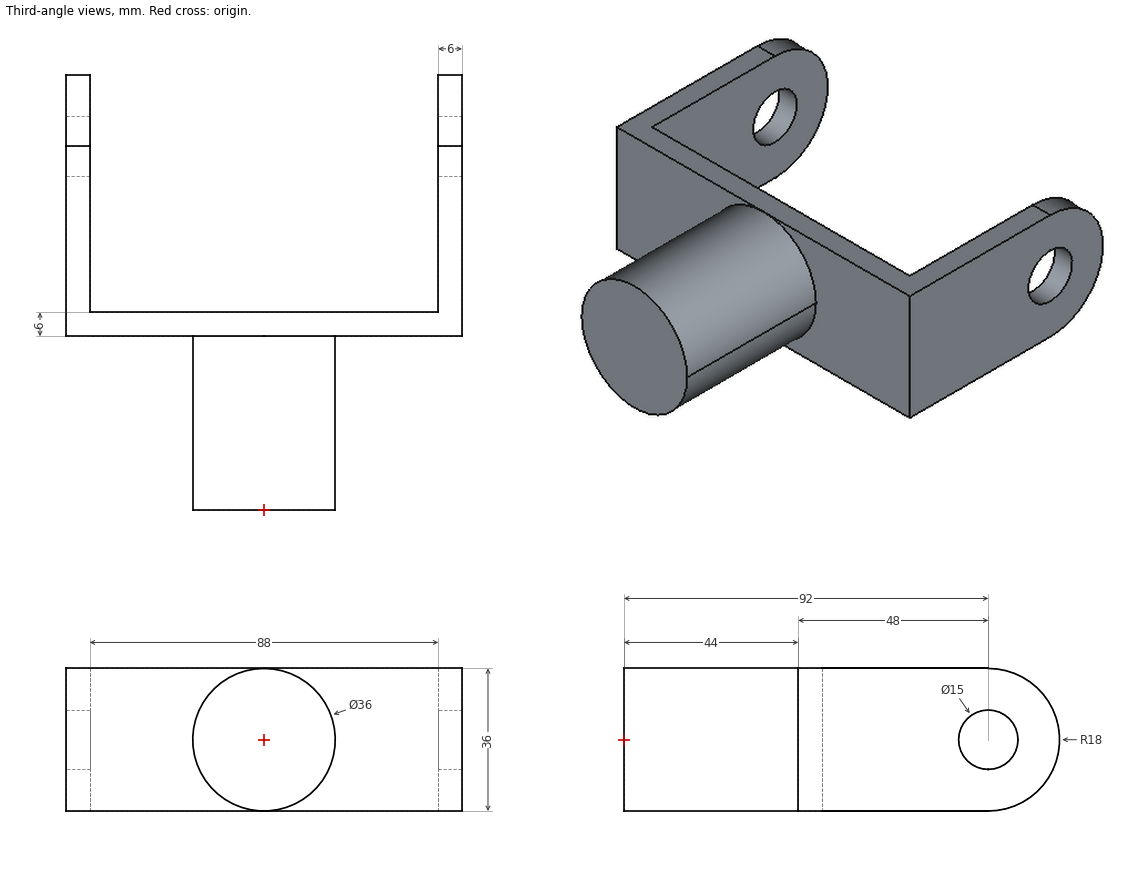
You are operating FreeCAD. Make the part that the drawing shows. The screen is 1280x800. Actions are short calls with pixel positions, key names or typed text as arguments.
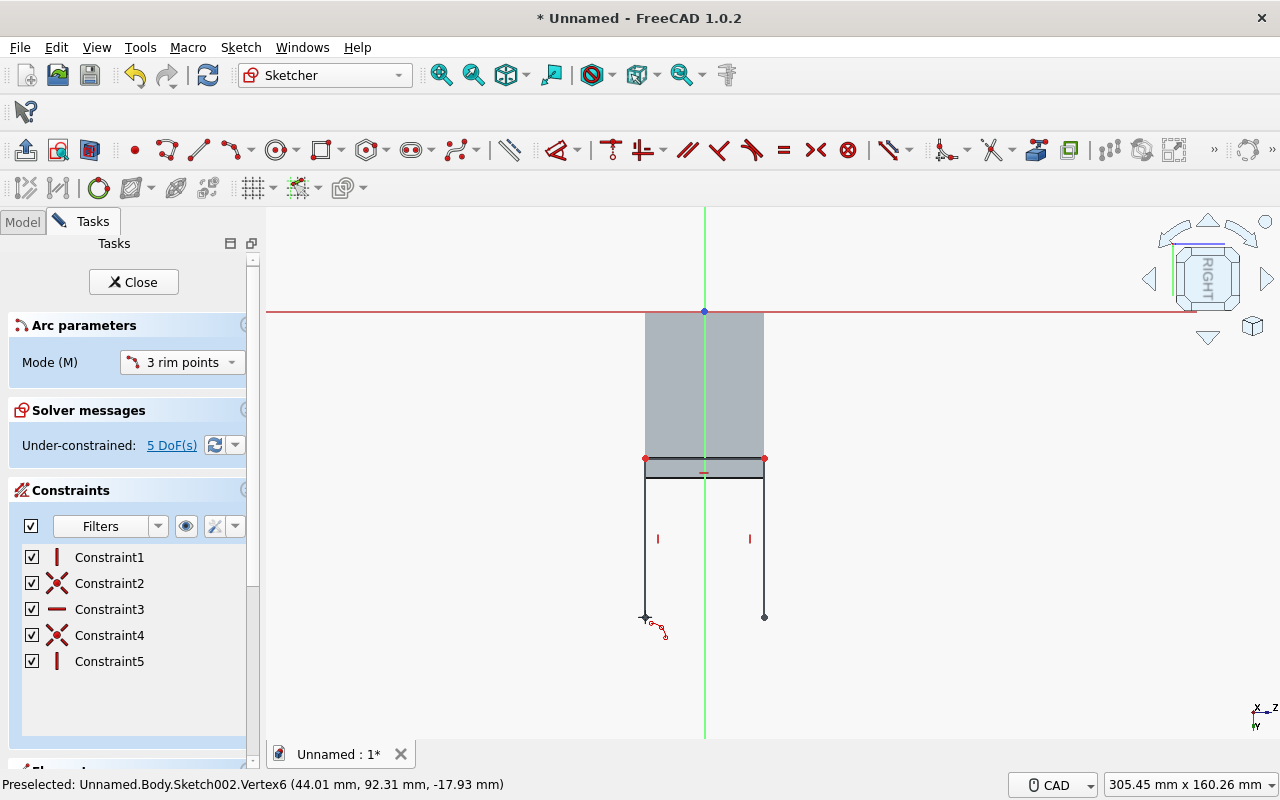
click(645, 618)
click(764, 618)
click(686, 674)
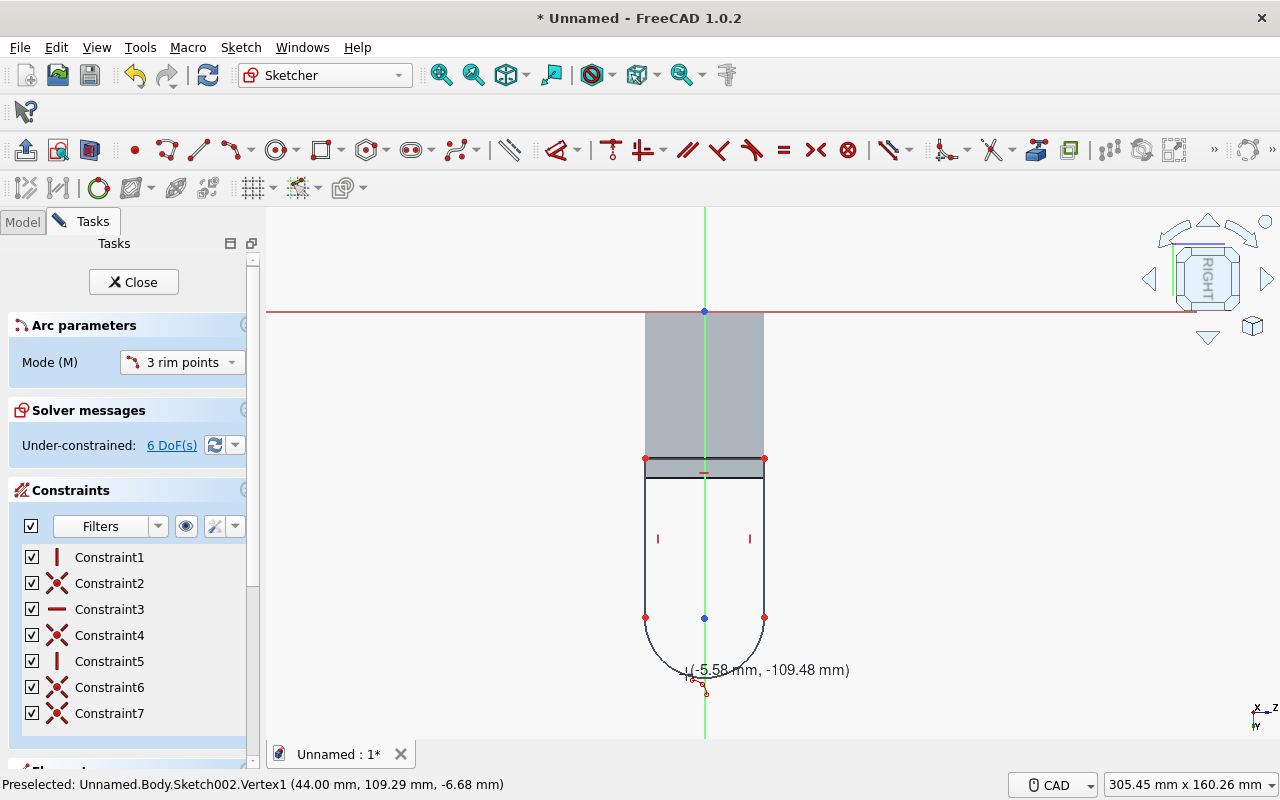
click(276, 150)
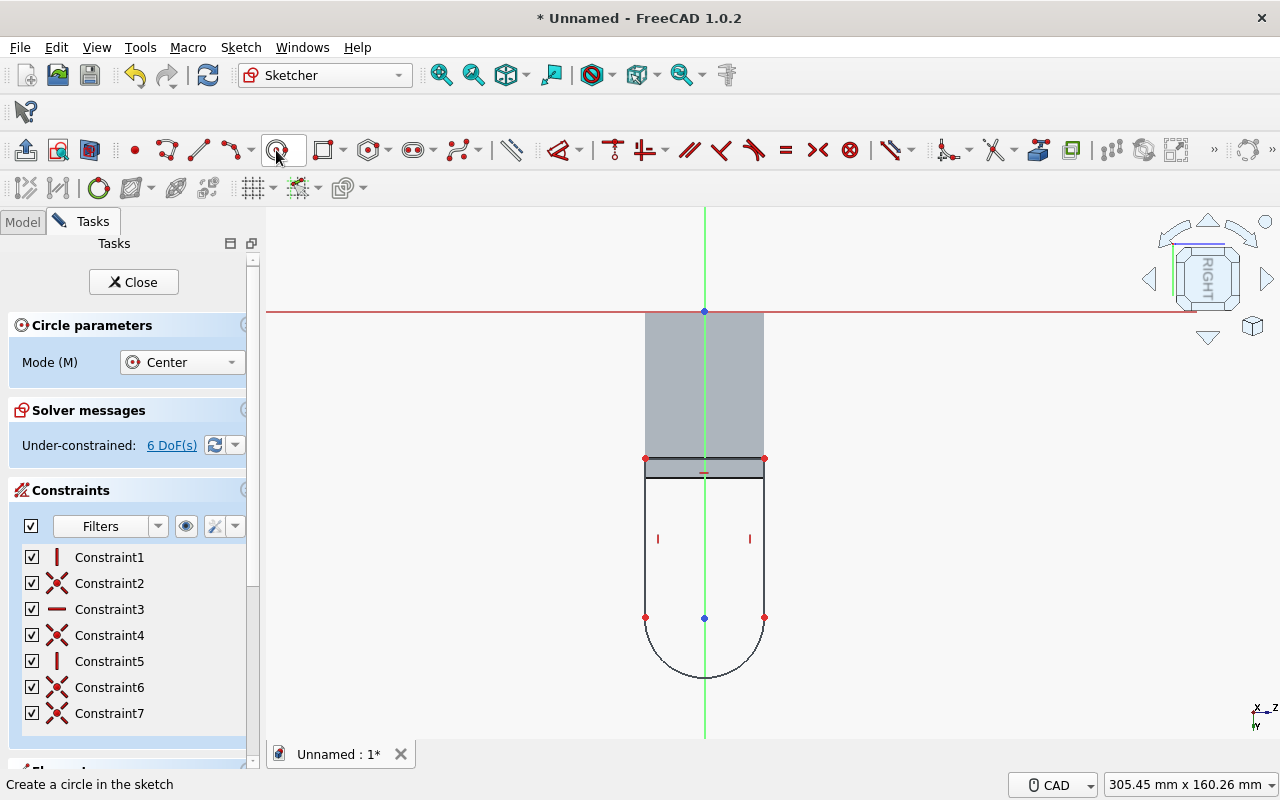
click(705, 617)
click(722, 599)
key(Escape)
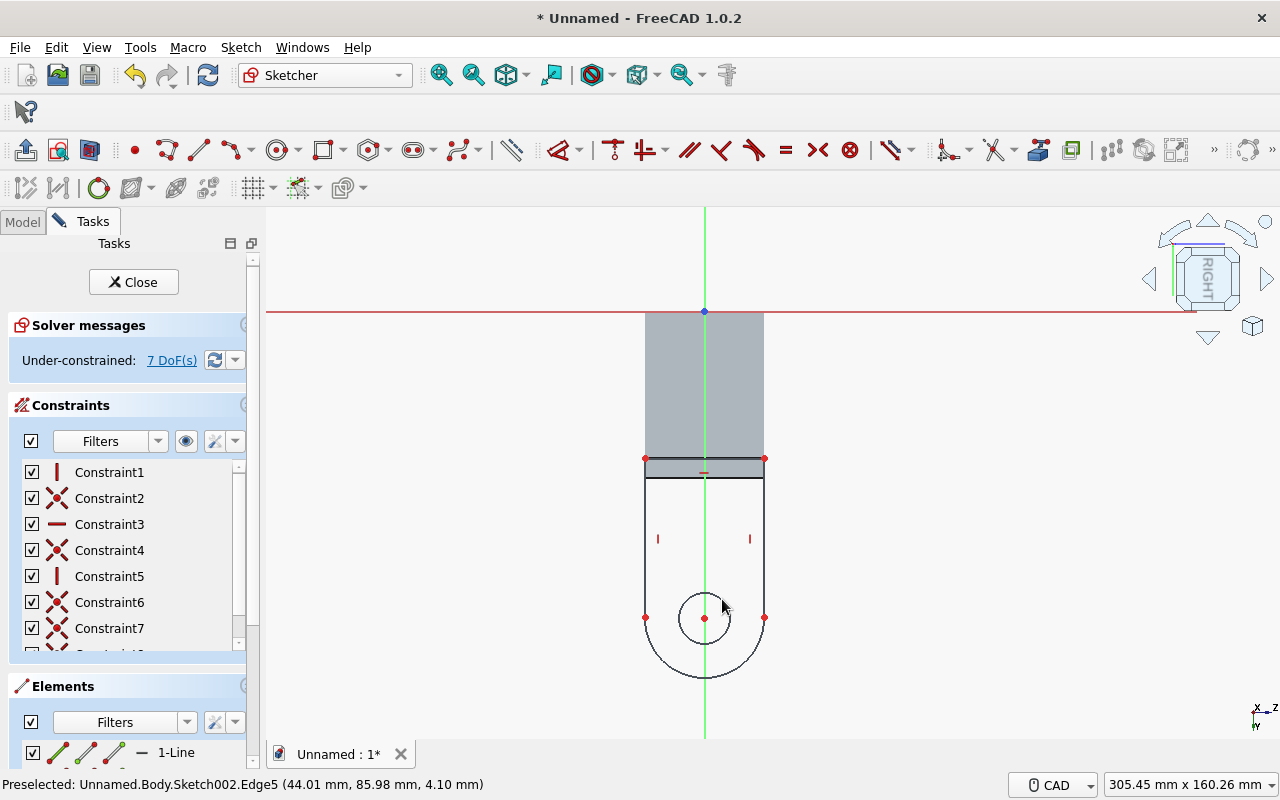
click(764, 570)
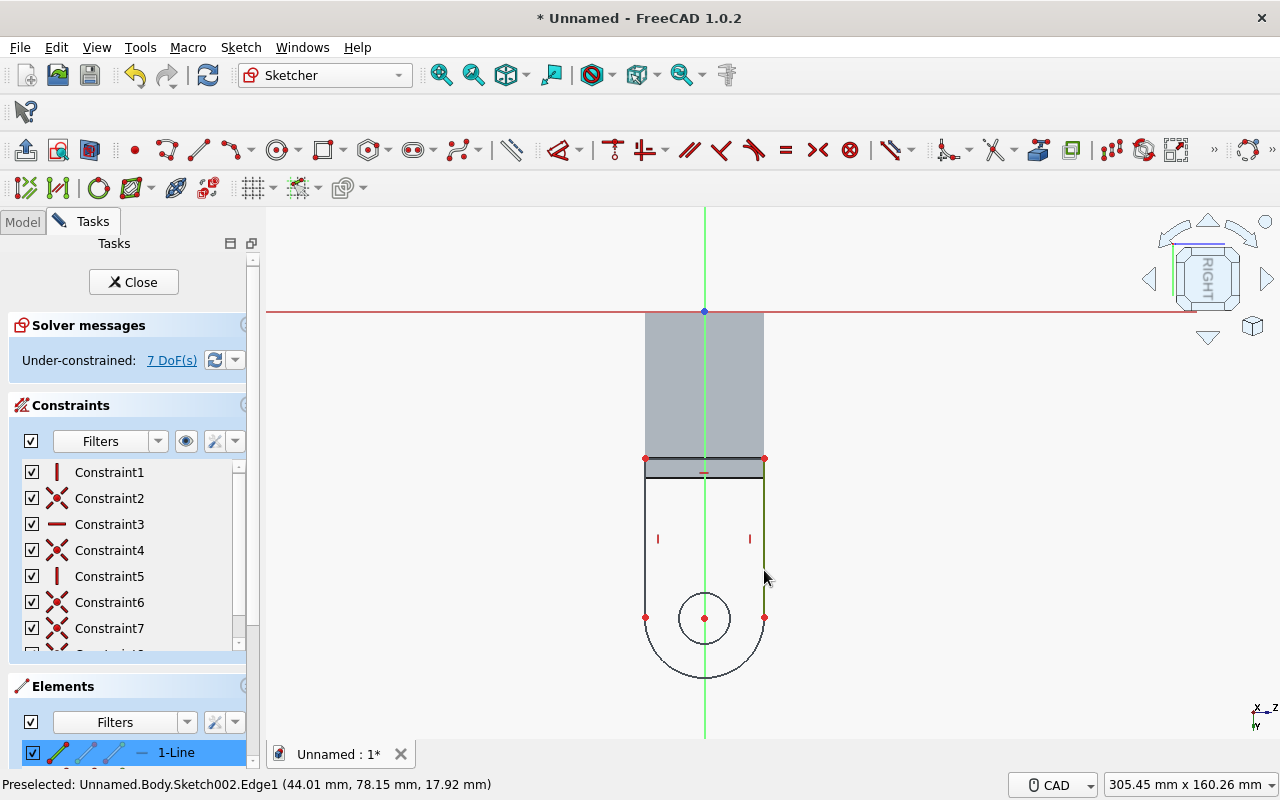
click(669, 666)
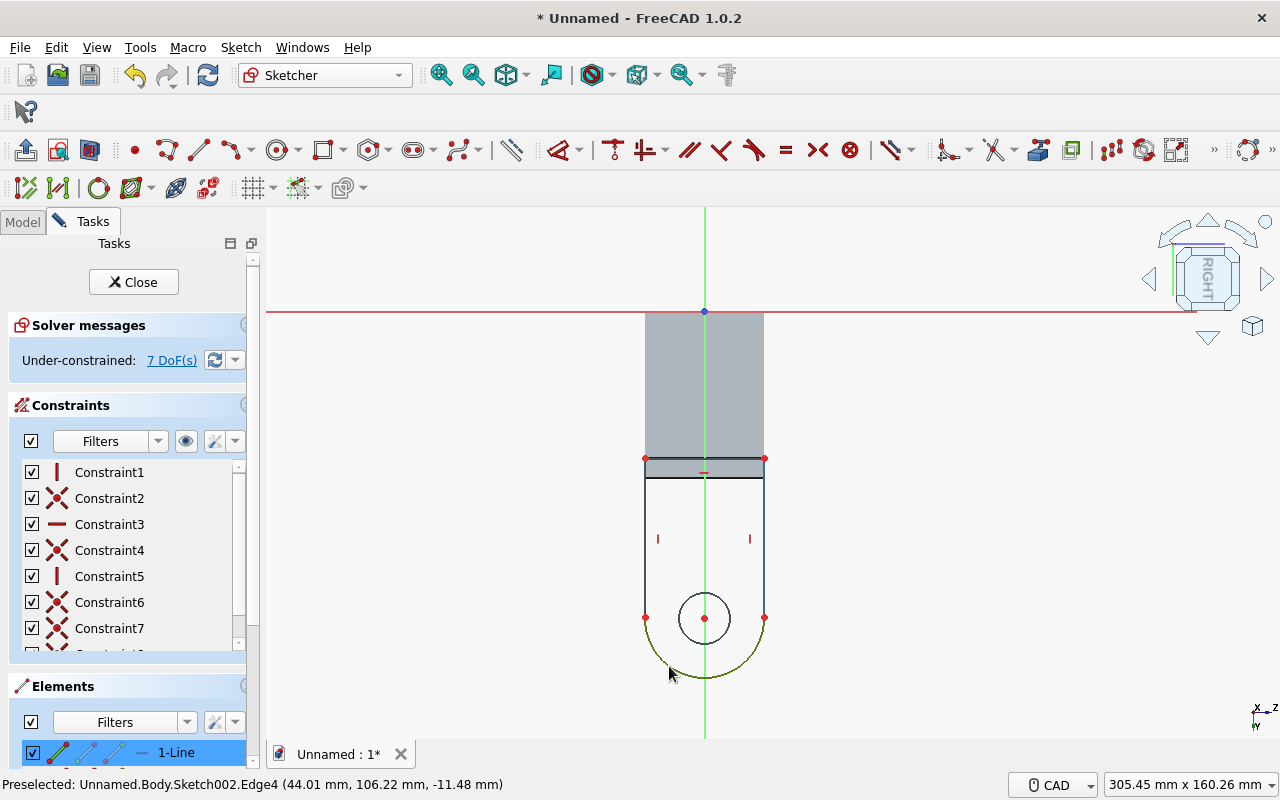
key(t)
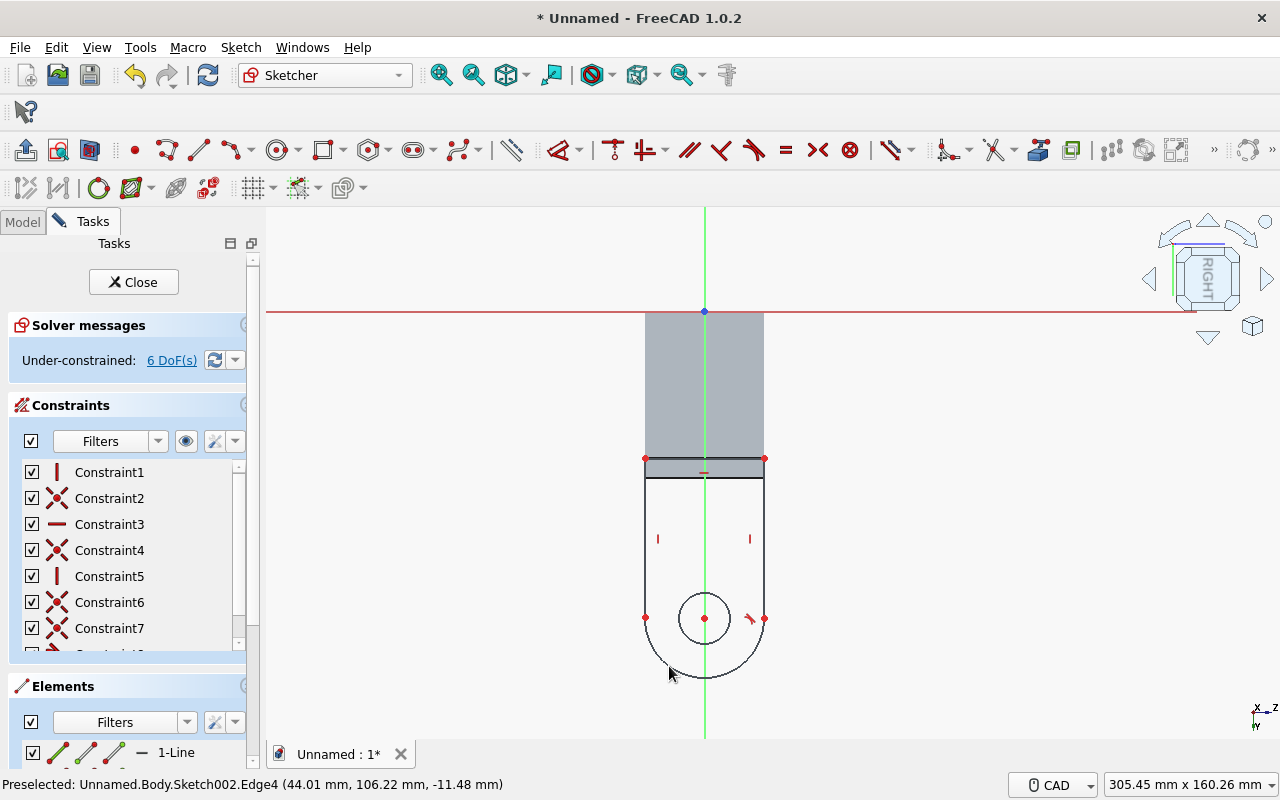
click(645, 507)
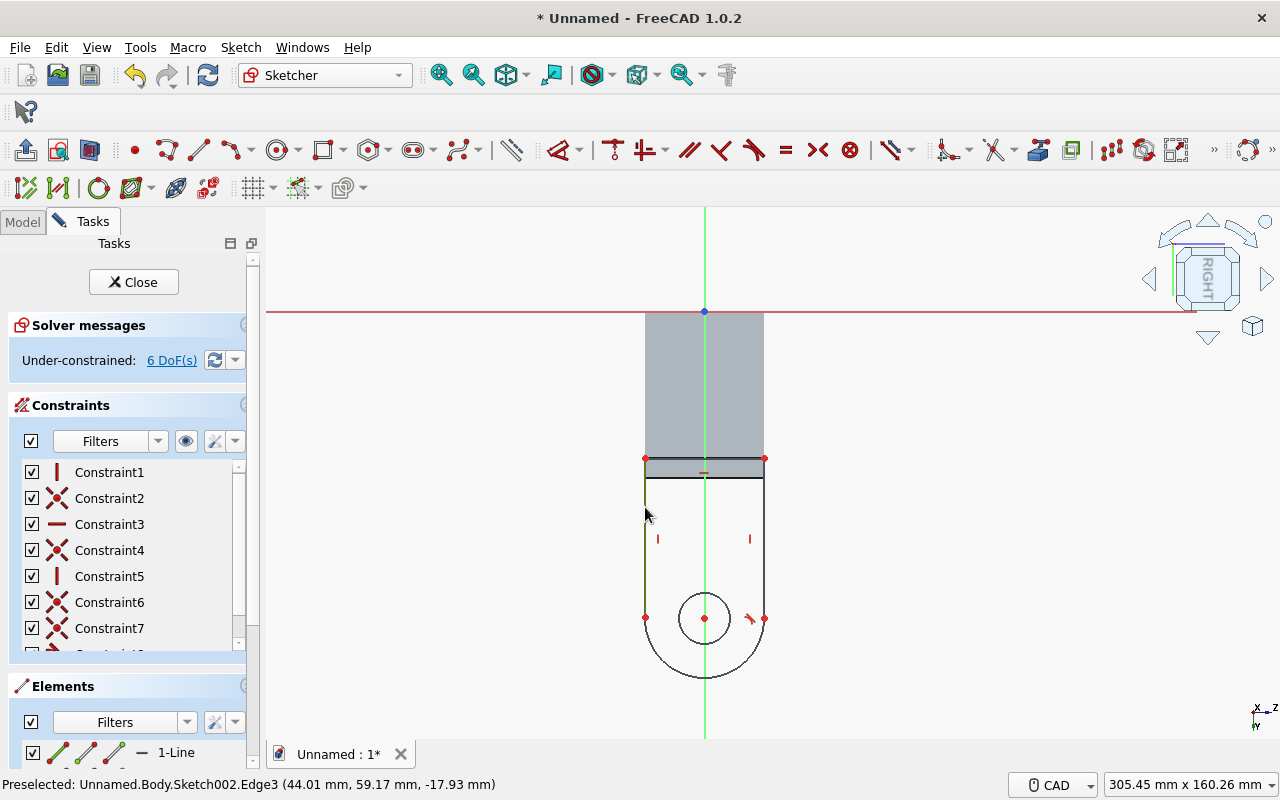
click(669, 666)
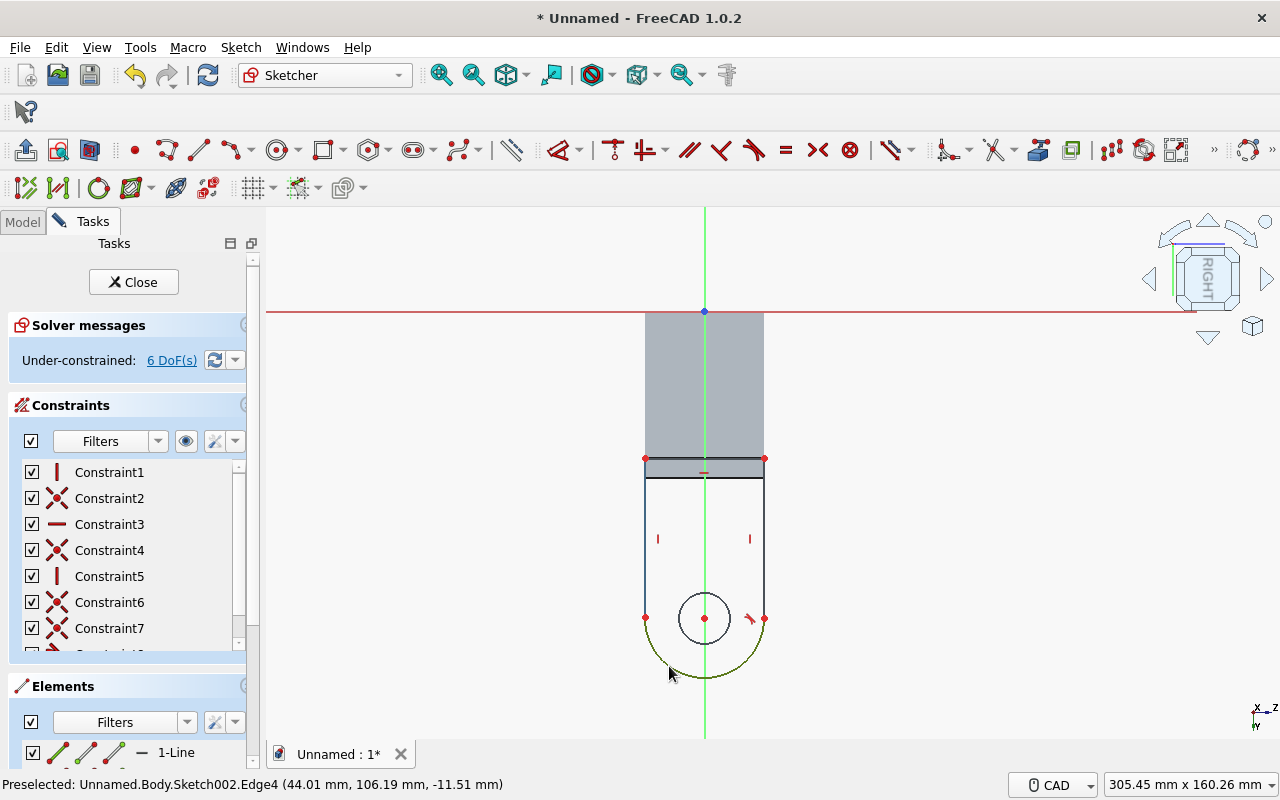
key(t)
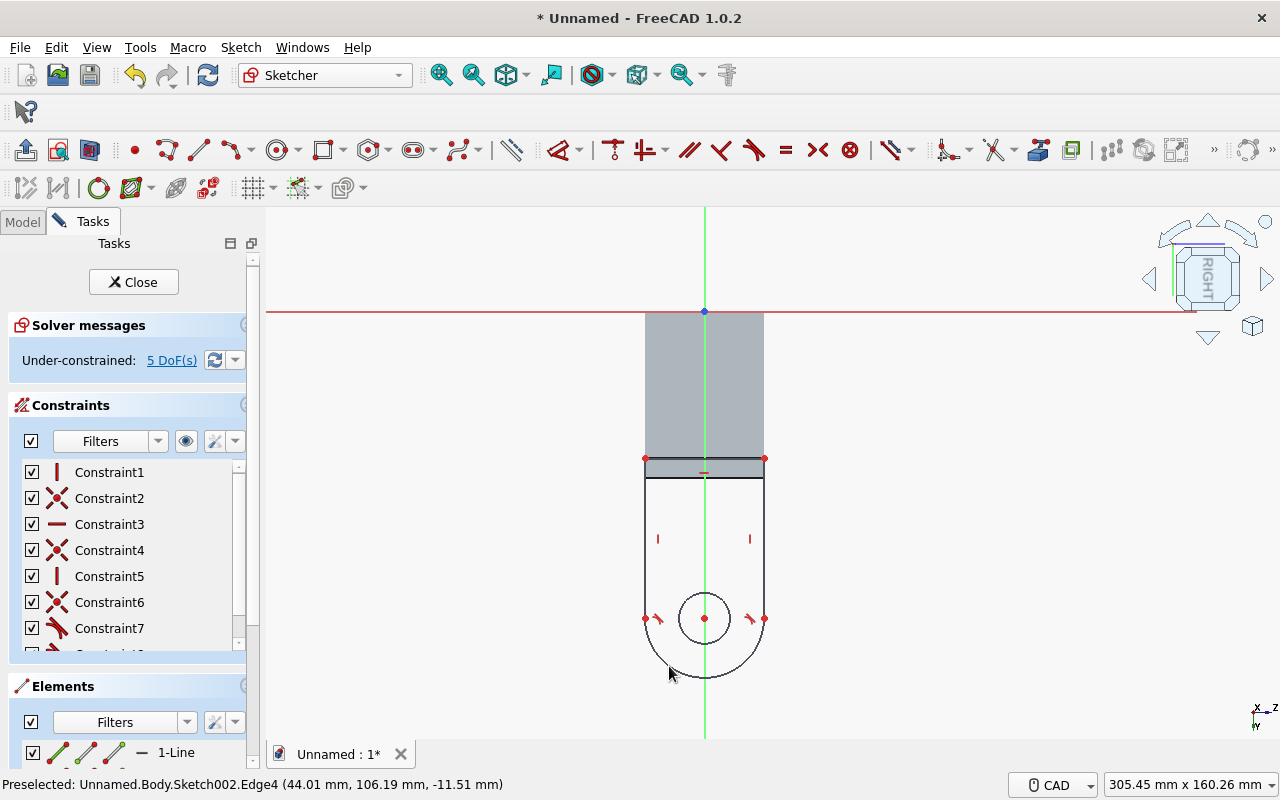
click(705, 618)